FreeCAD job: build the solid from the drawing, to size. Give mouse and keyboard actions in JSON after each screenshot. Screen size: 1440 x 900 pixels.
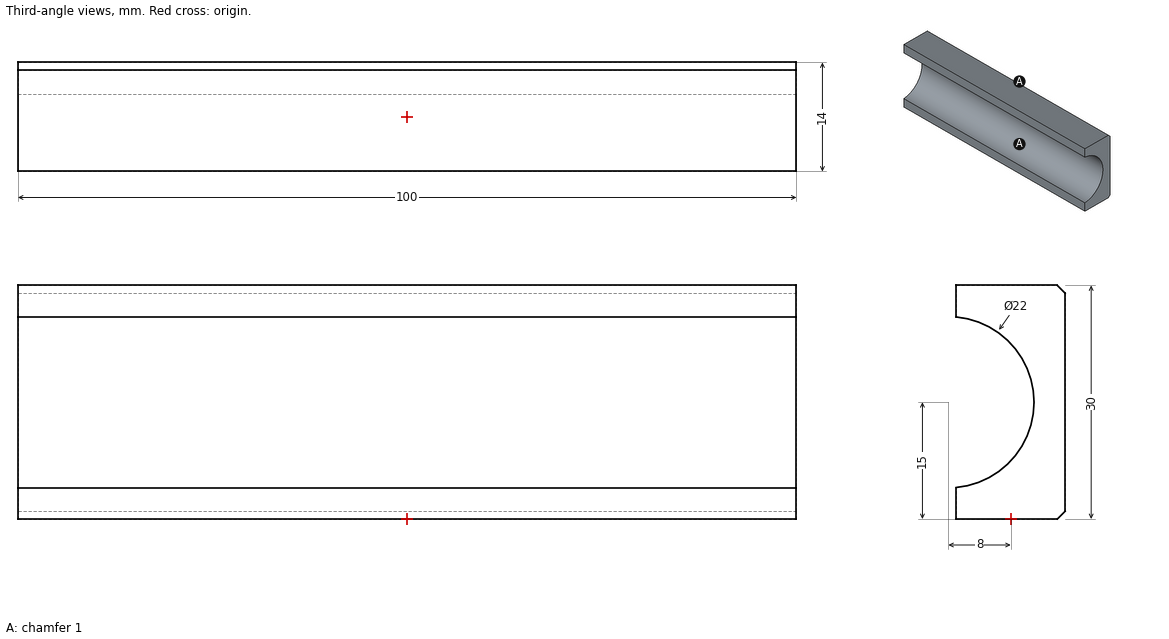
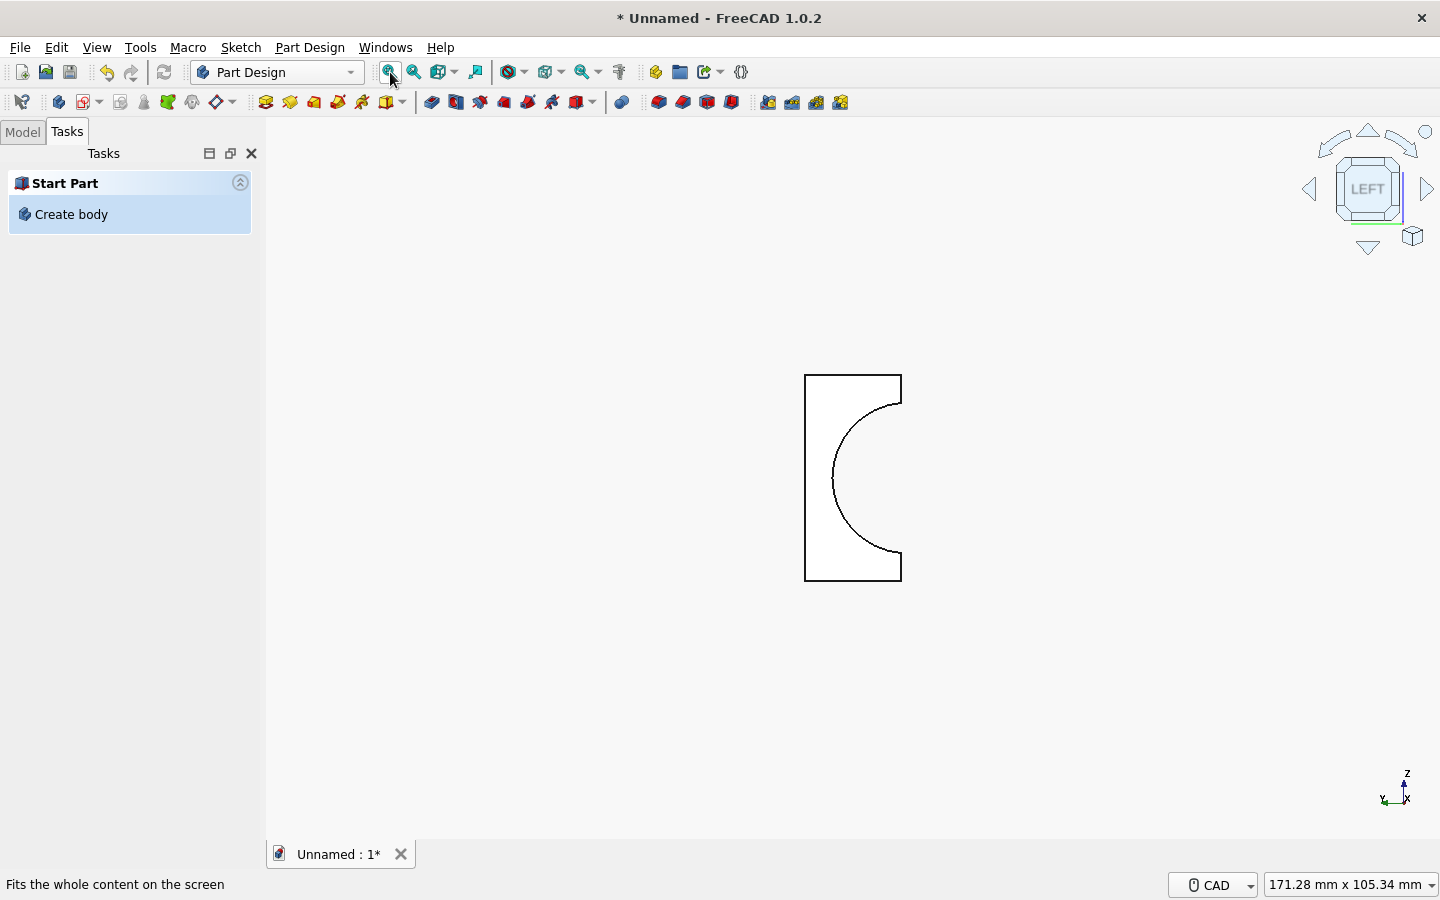
{"action": "key", "text": "0"}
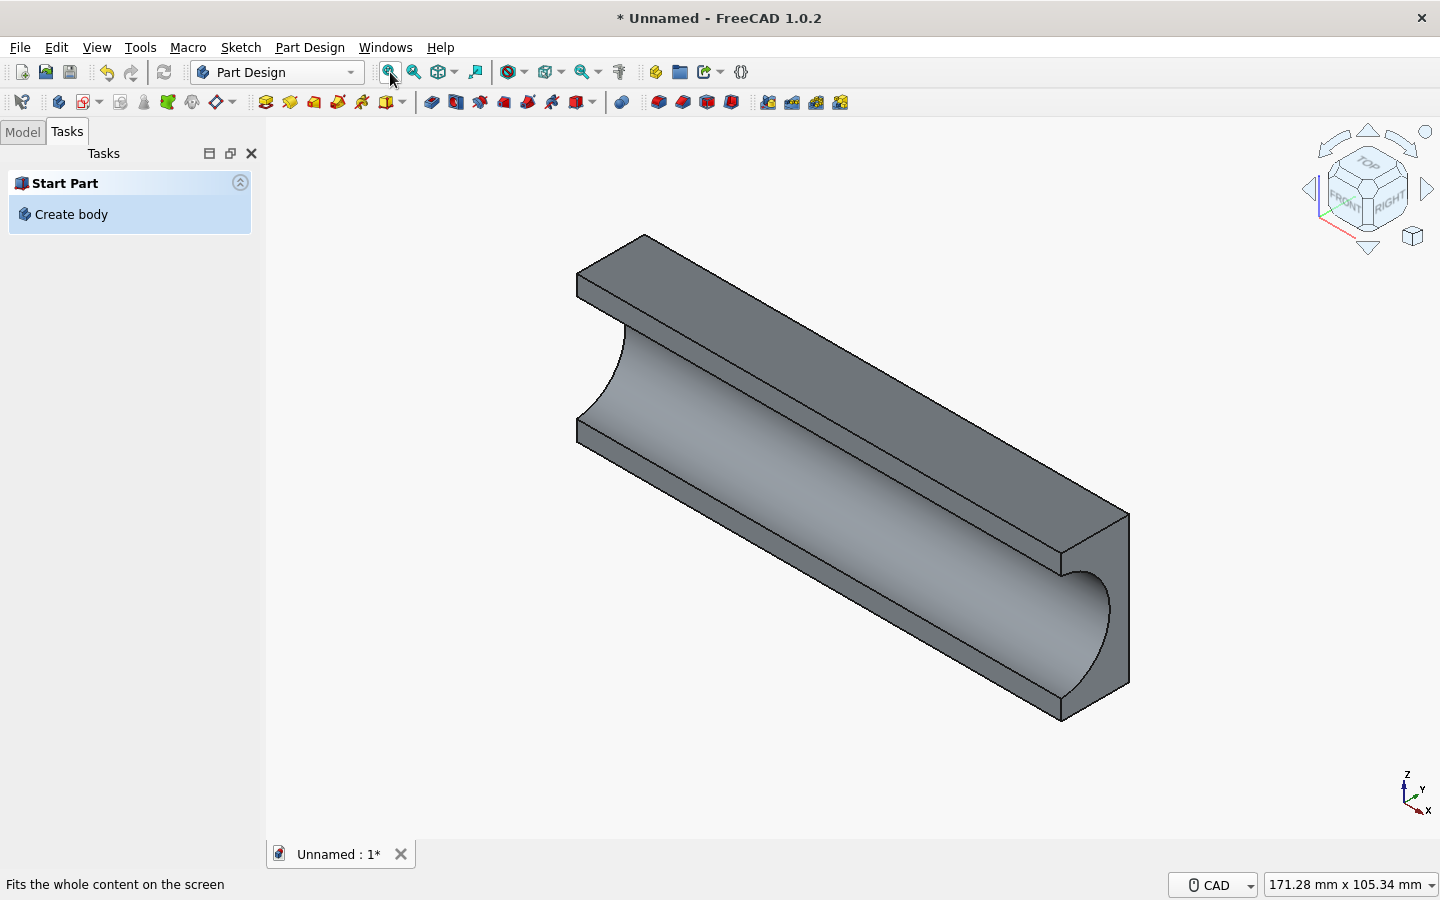
{"action": "key", "text": "2"}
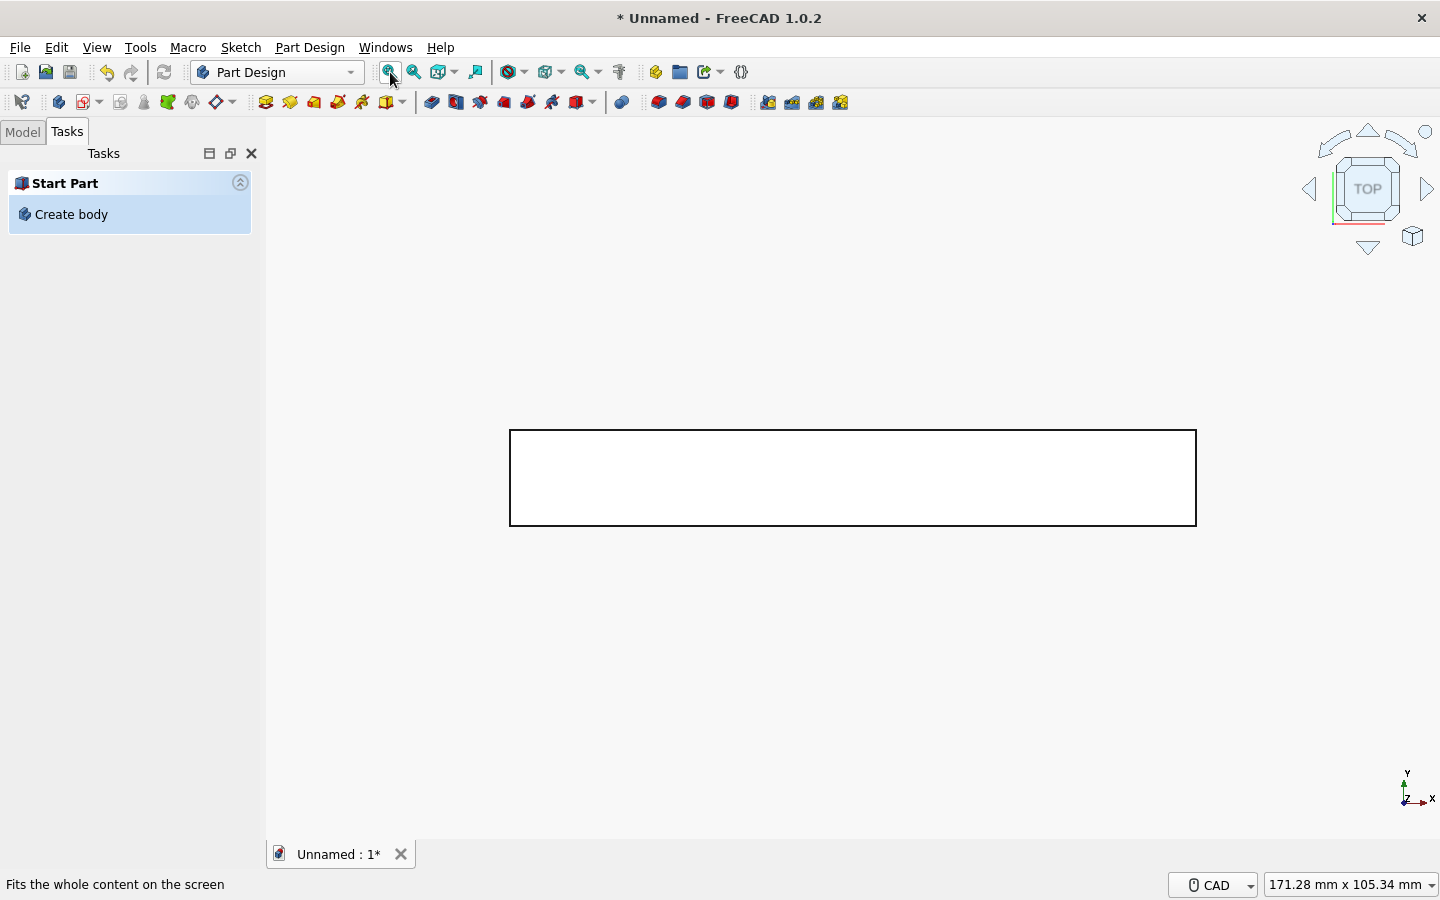
{"action": "left_click", "coordinate": [853, 429]}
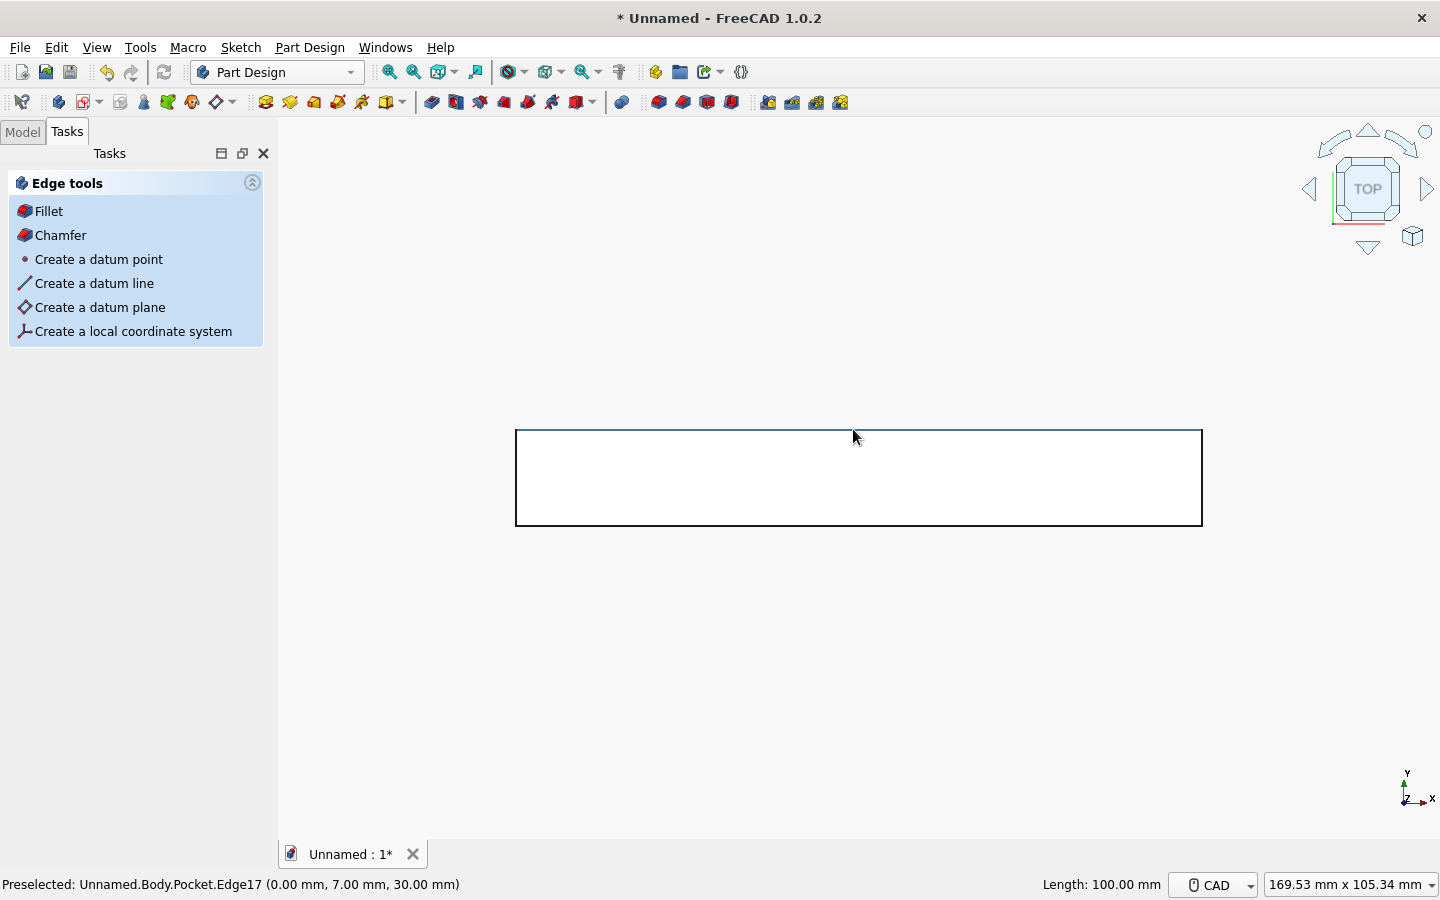
{"action": "key", "text": "1"}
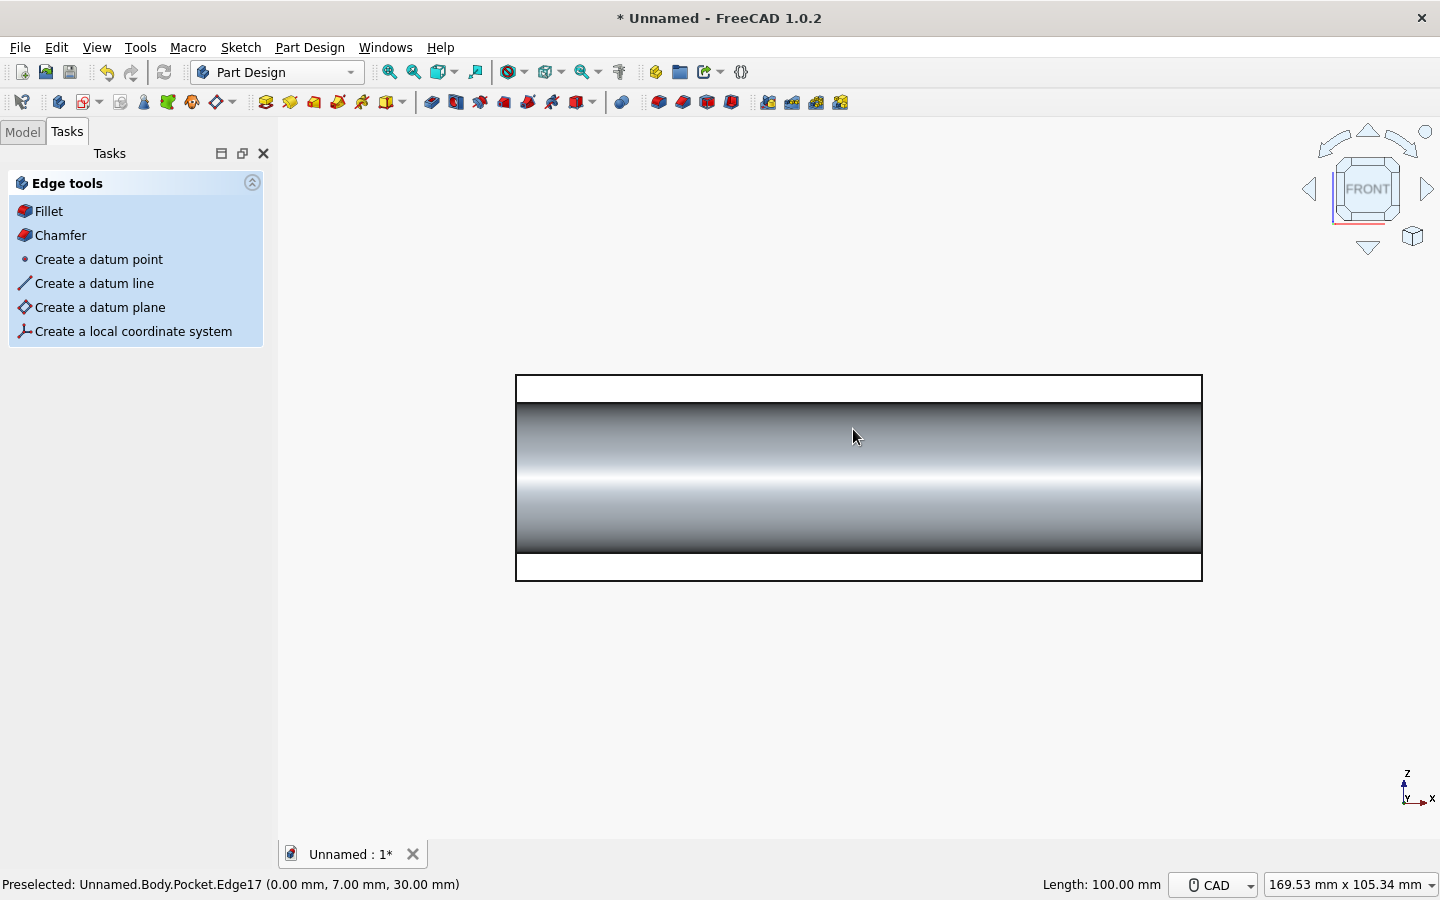
{"action": "key", "text": "3"}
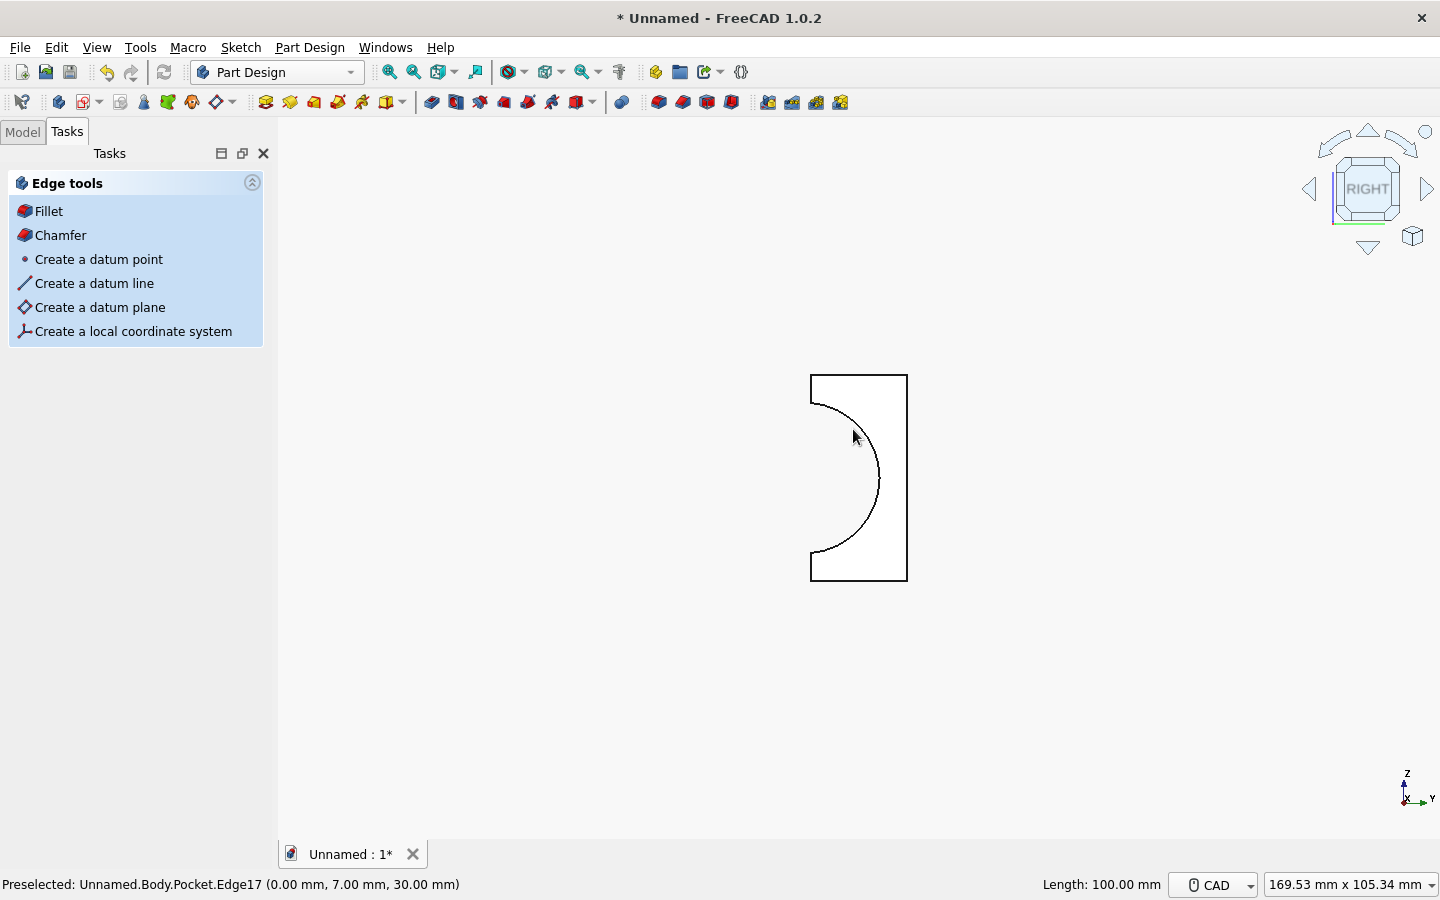
{"action": "key", "text": "v f"}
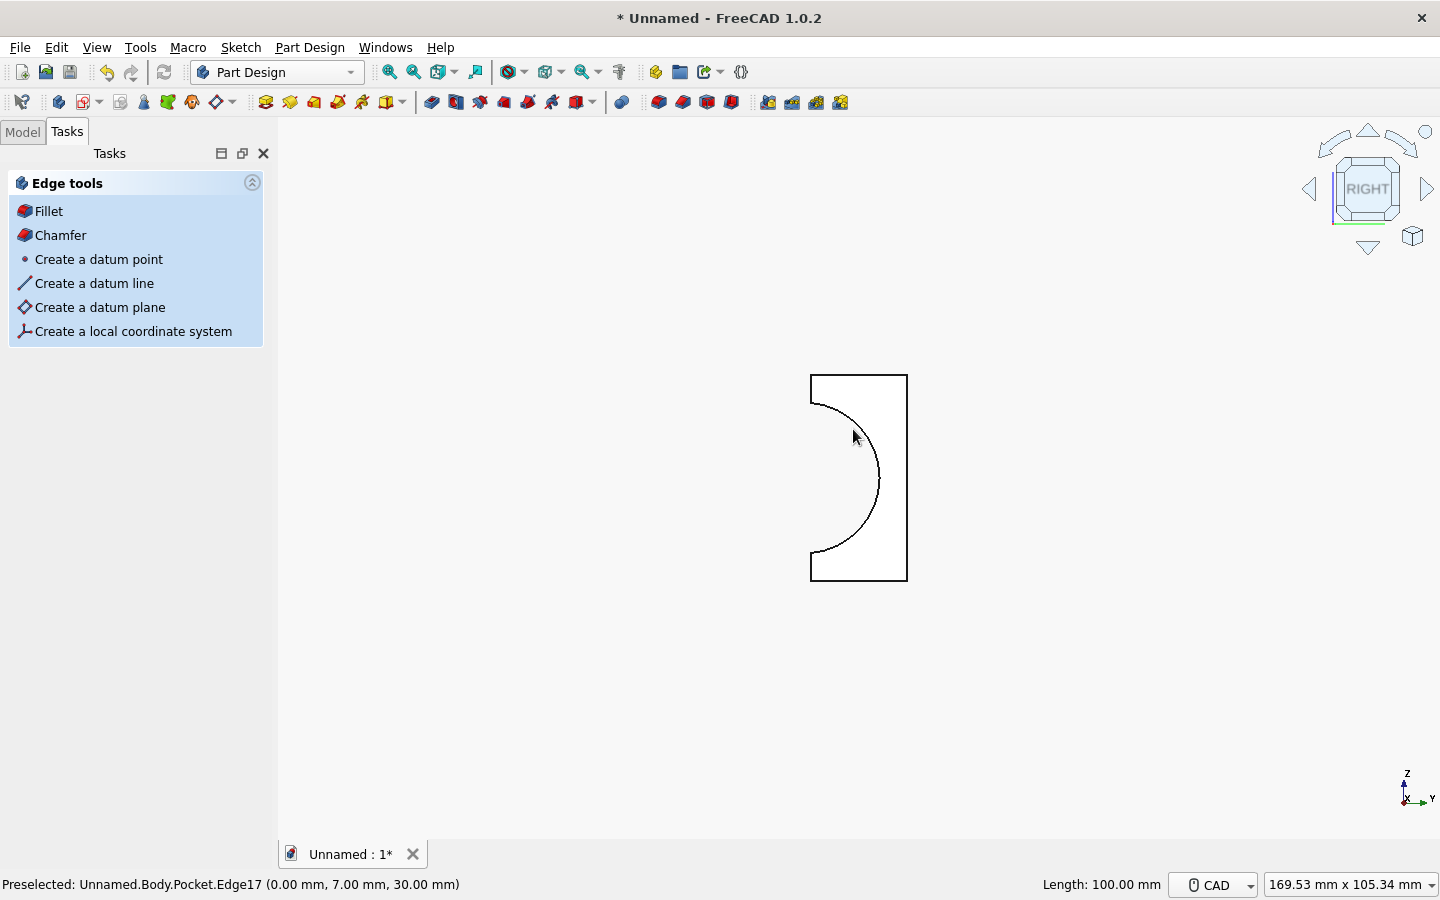
{"action": "key", "text": "5"}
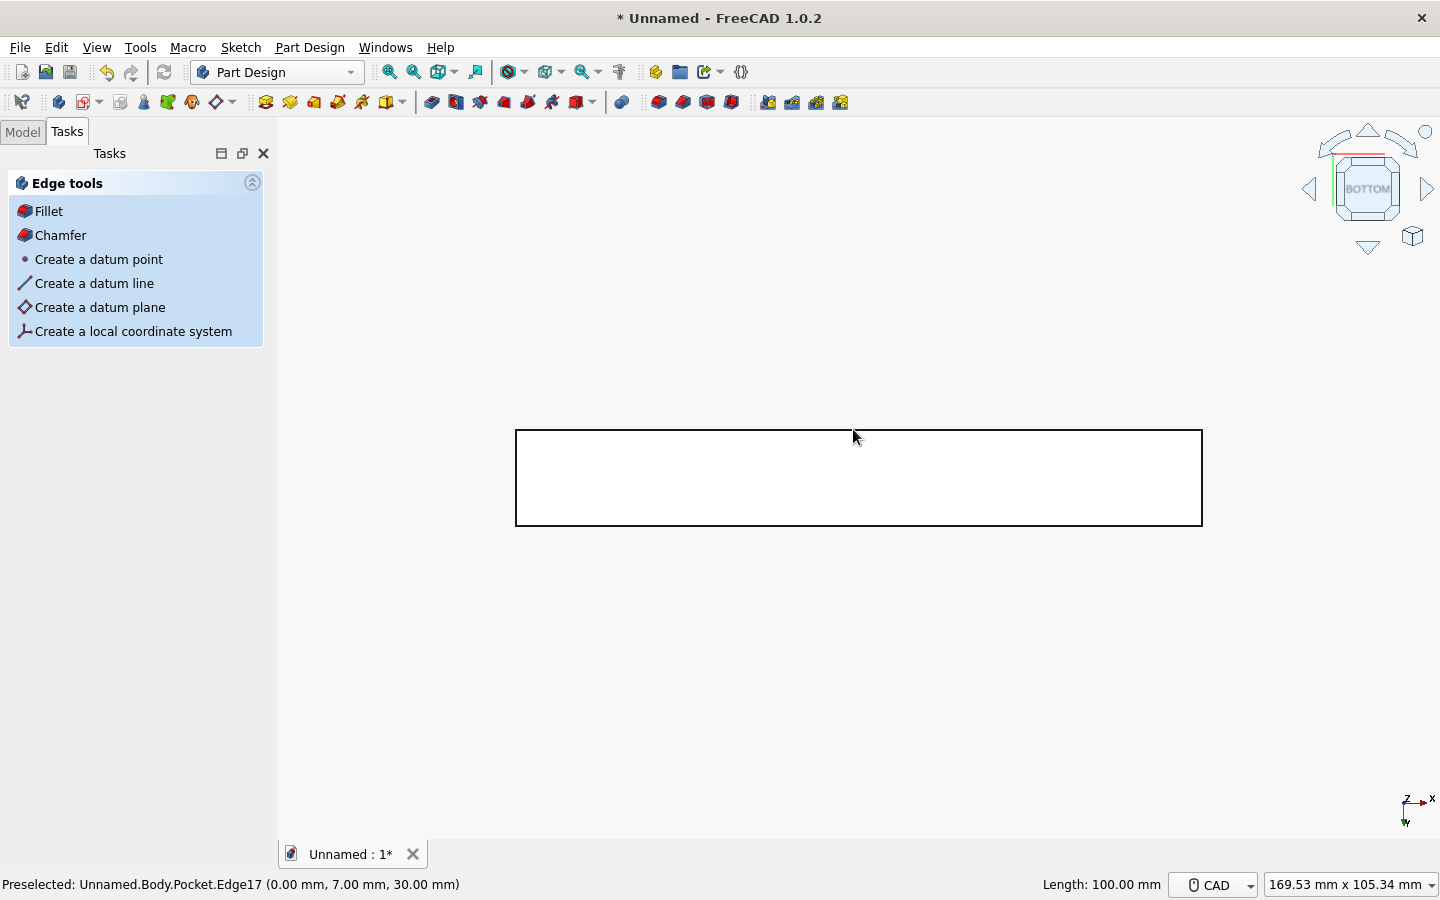
{"action": "left_click", "coordinate": [859, 525], "text": "ctrl"}